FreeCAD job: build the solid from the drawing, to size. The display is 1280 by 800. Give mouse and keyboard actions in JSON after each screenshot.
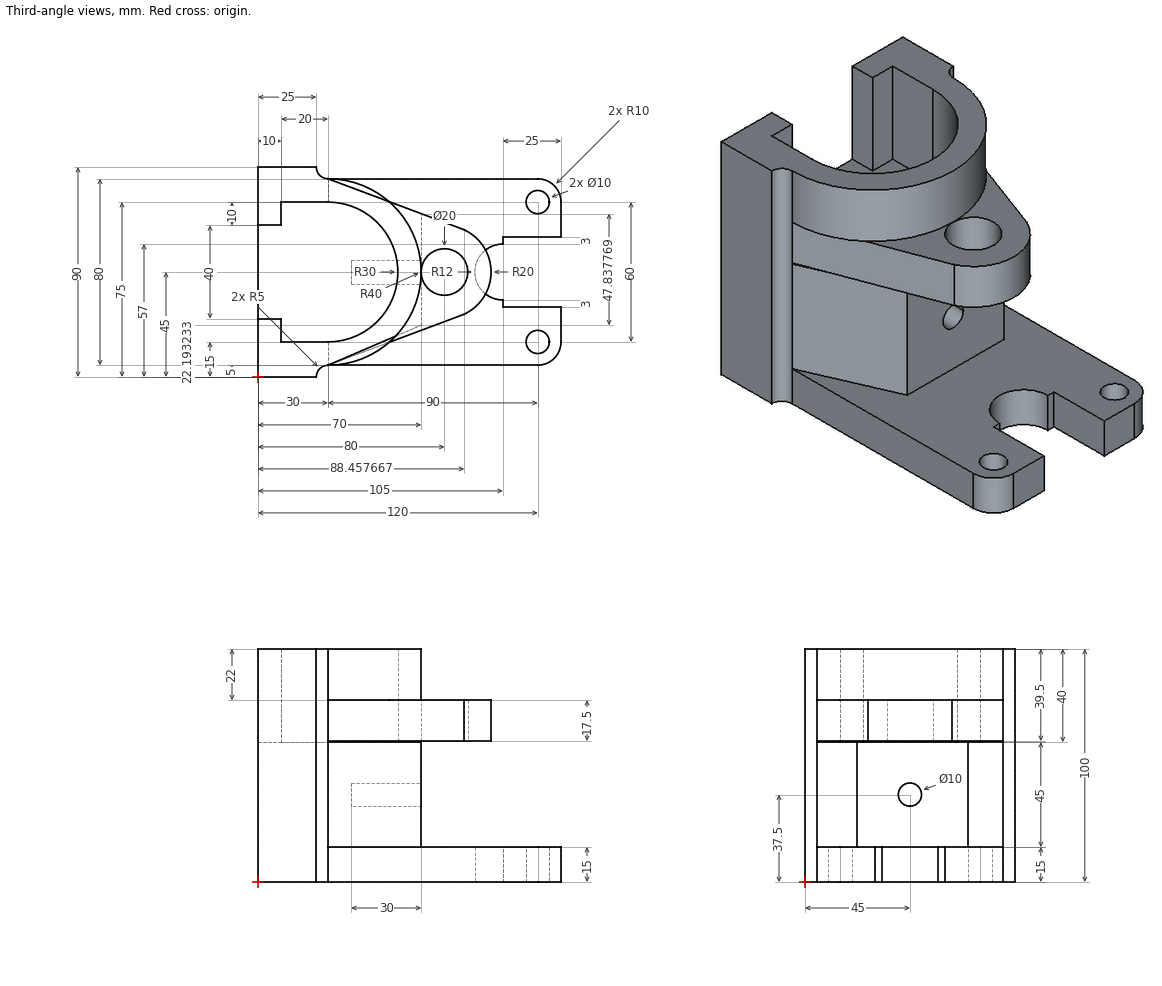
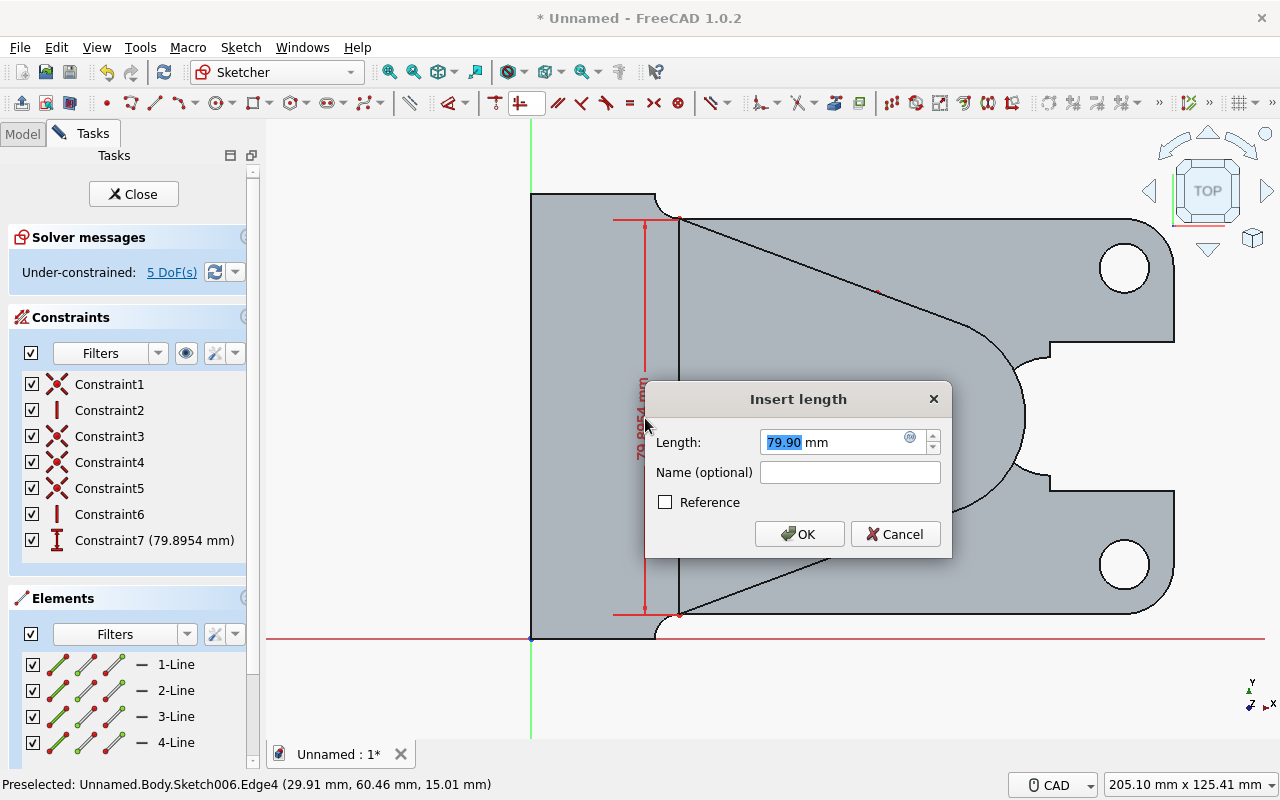
{"action": "type", "text": "80"}
{"action": "key", "text": "Return"}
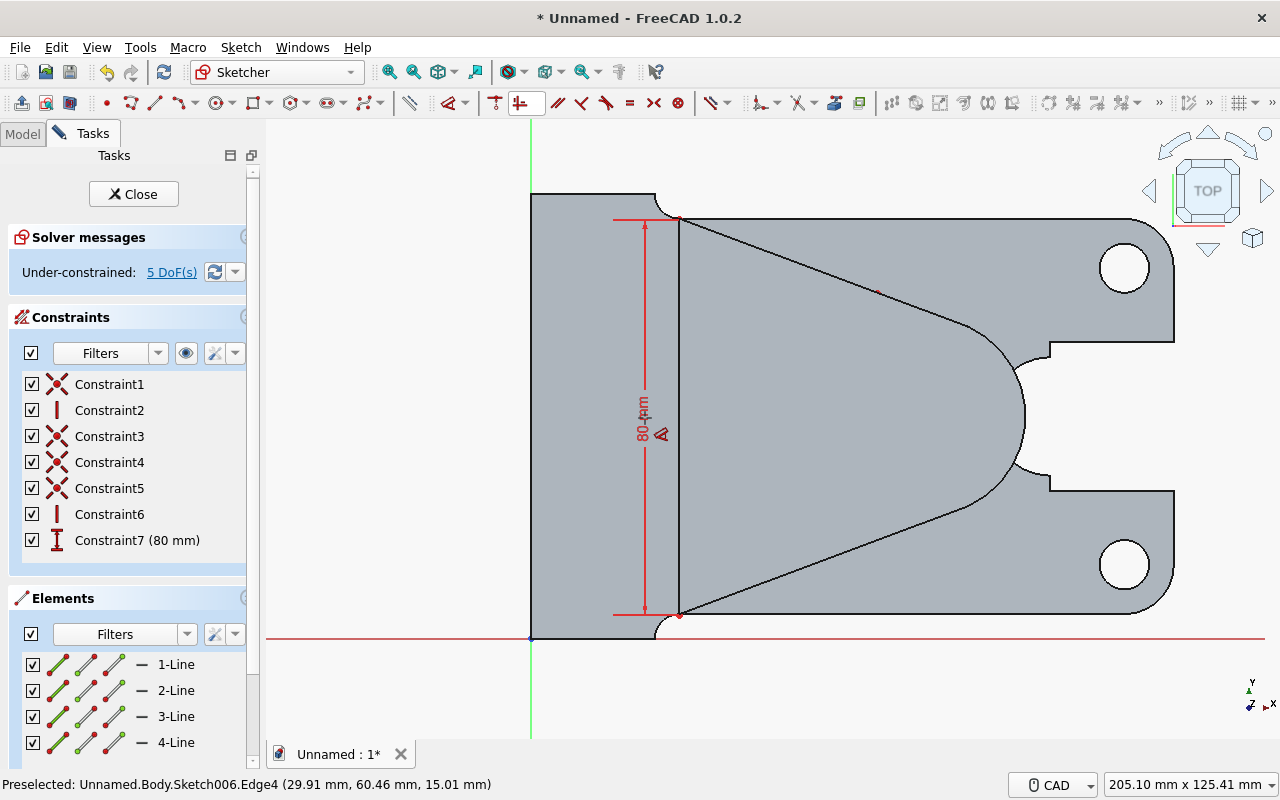
{"action": "scroll", "coordinate": [679, 615], "scroll_direction": "up", "scroll_amount": 3}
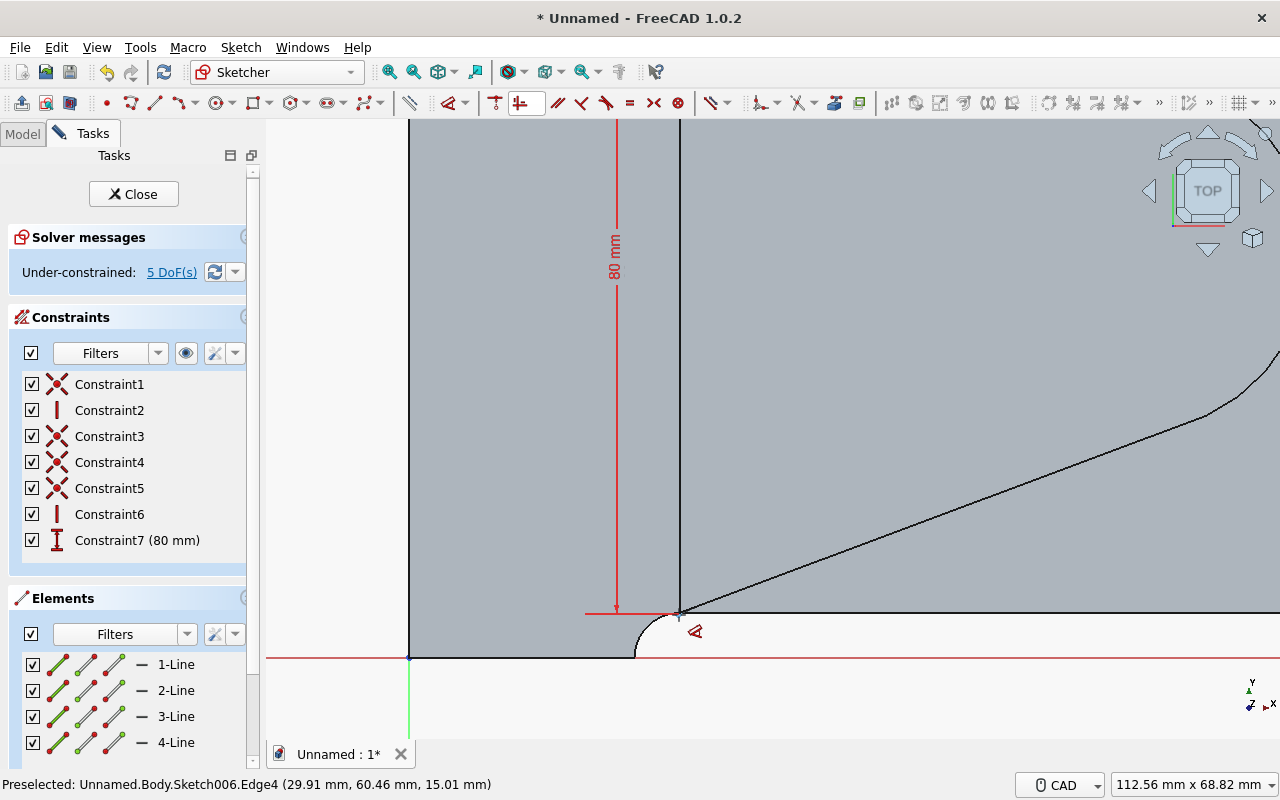
{"action": "left_click", "coordinate": [679, 614]}
{"action": "left_click", "coordinate": [375, 636]}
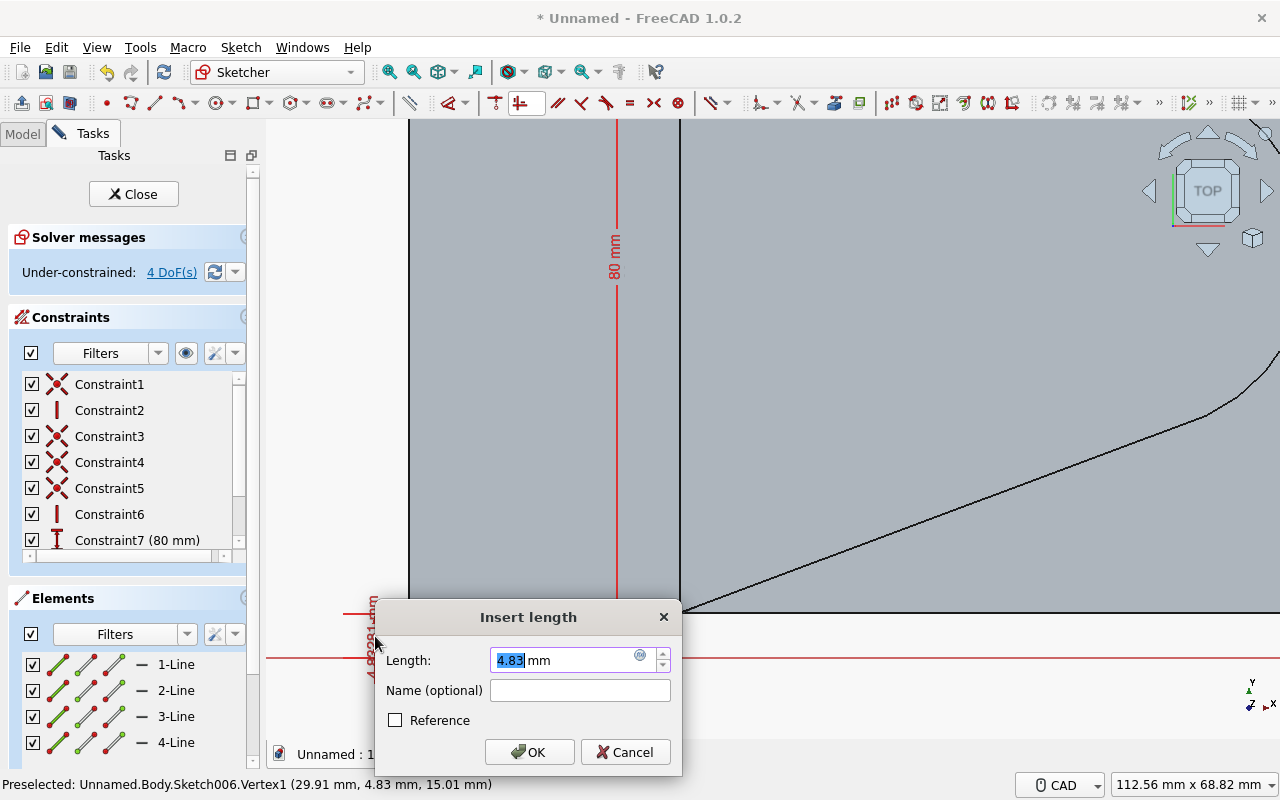
{"action": "type", "text": "5"}
{"action": "key", "text": "Return"}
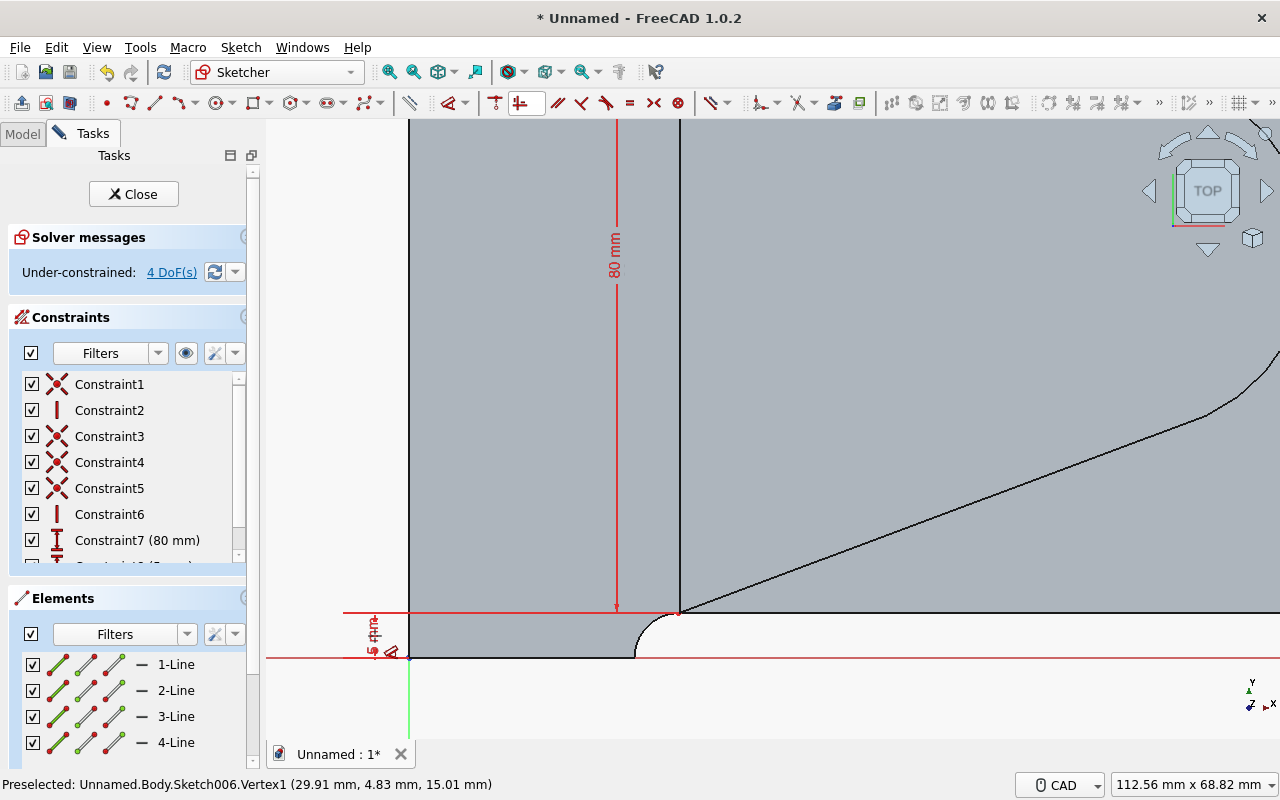
{"action": "left_click", "coordinate": [679, 613]}
{"action": "left_click", "coordinate": [544, 692]}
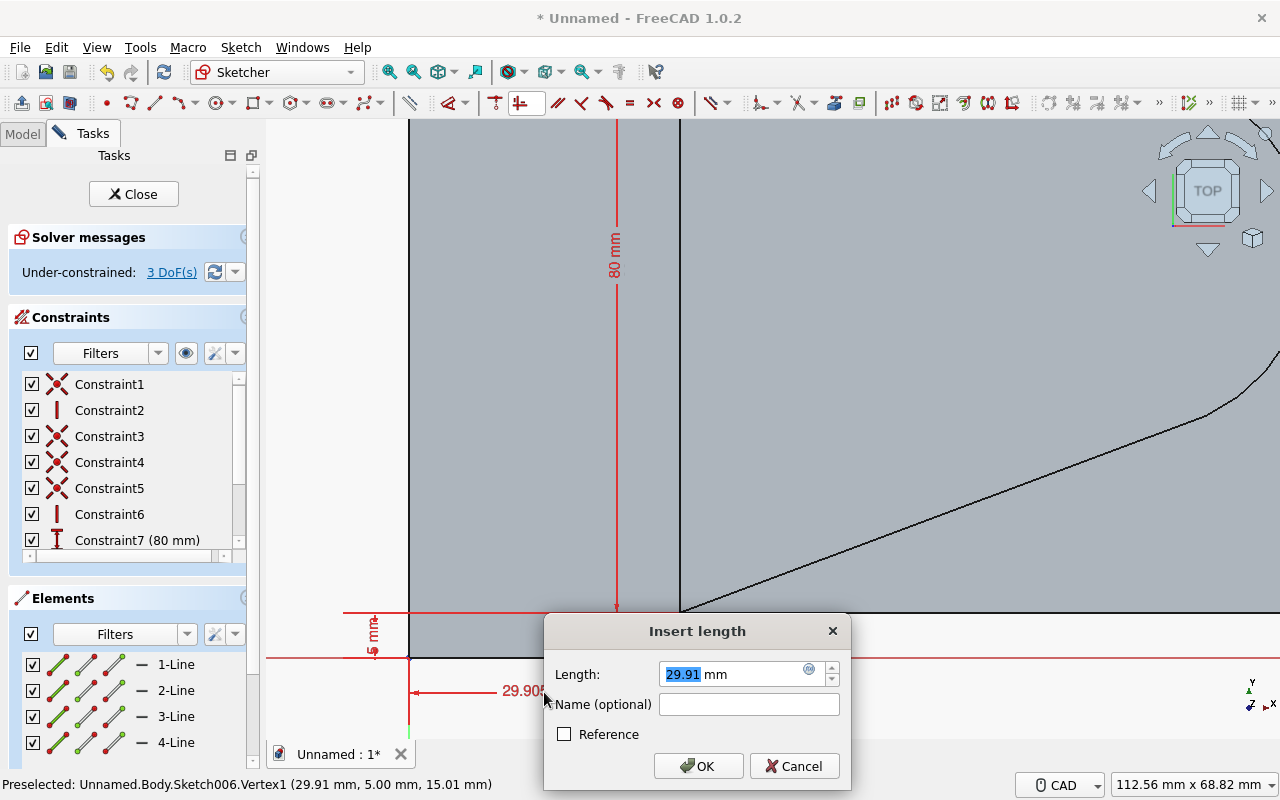
{"action": "type", "text": "30"}
{"action": "key", "text": "Return"}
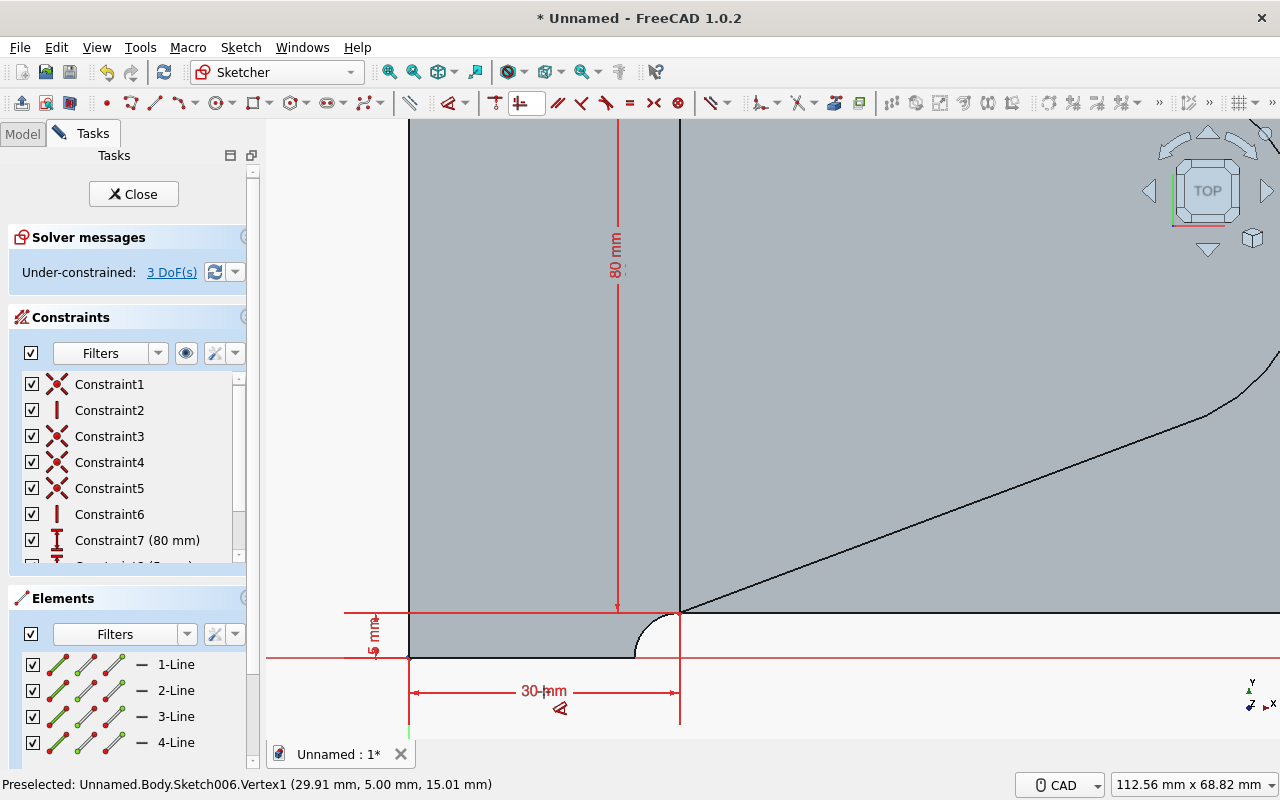
{"action": "left_click", "coordinate": [1039, 459]}
{"action": "left_click", "coordinate": [724, 692]}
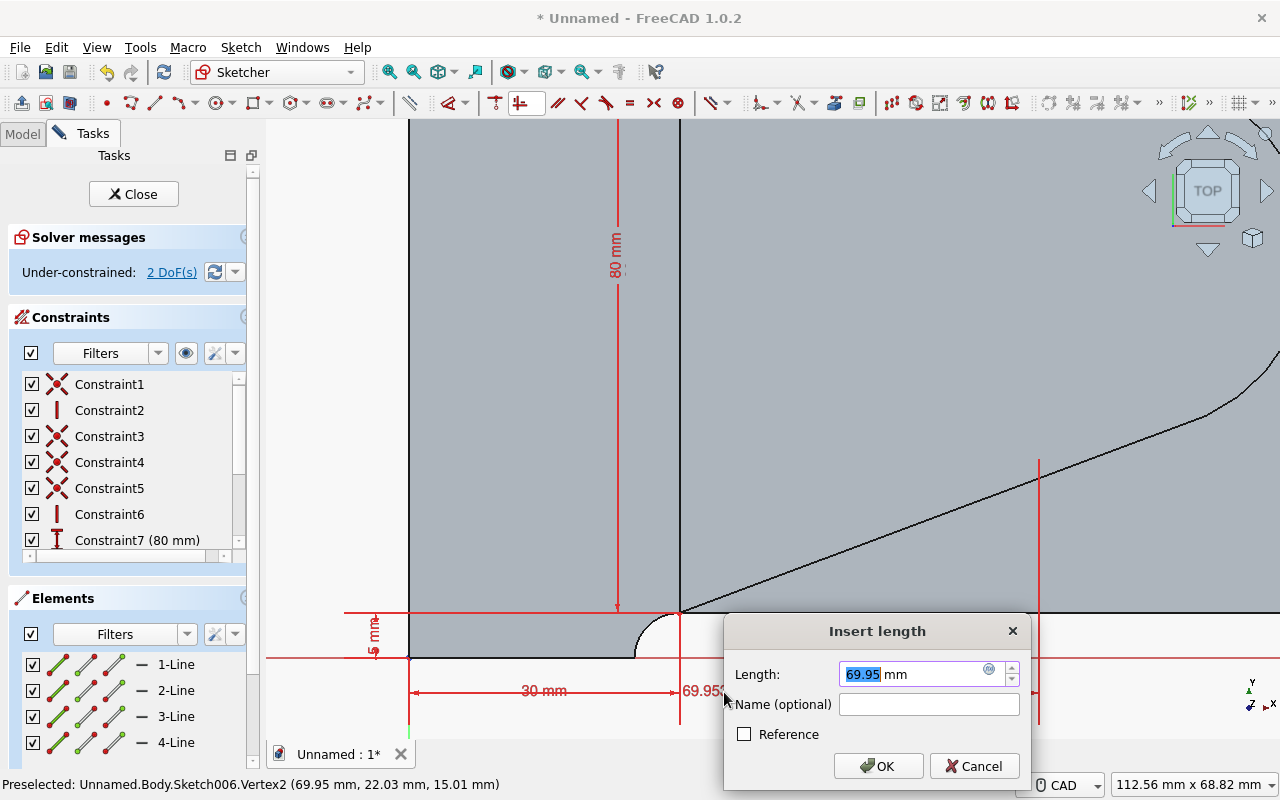
{"action": "type", "text": "70"}
{"action": "key", "text": "Return"}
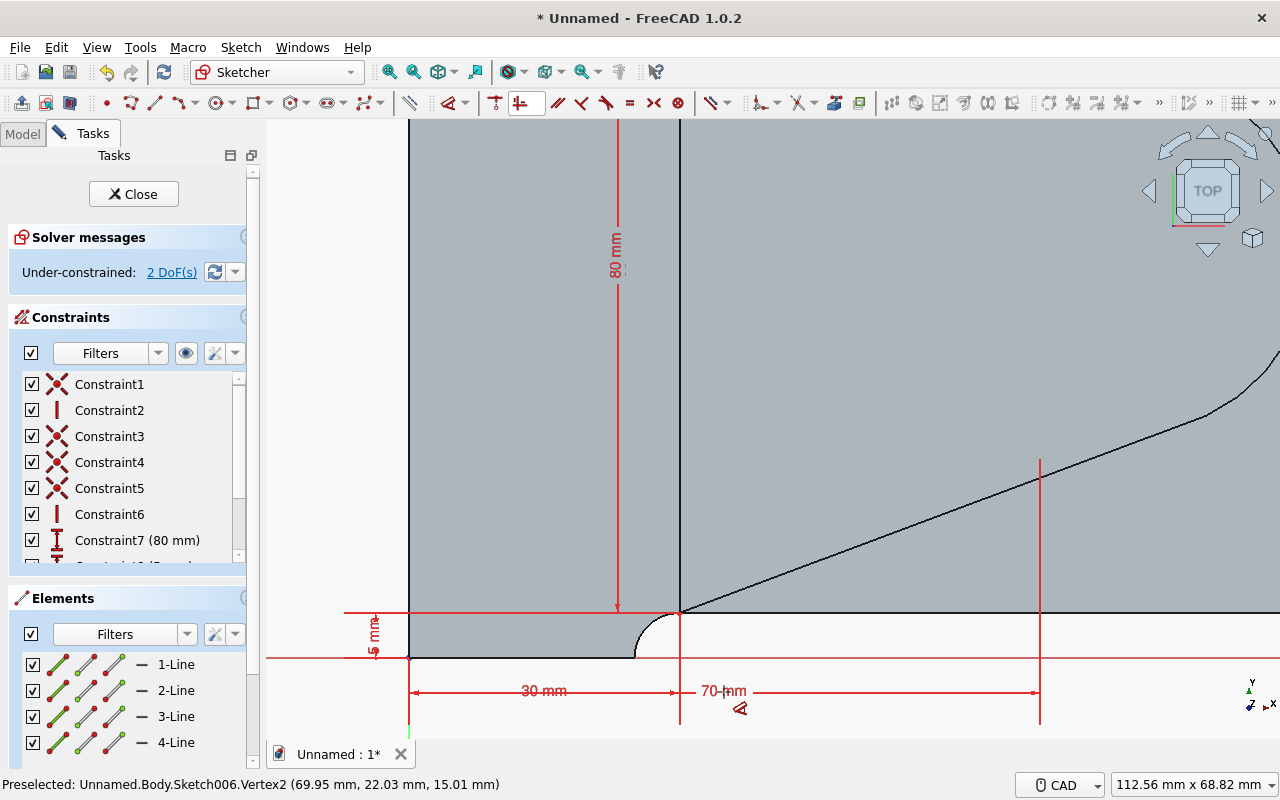
{"action": "left_click", "coordinate": [1040, 330]}
{"action": "left_click", "coordinate": [1074, 303]}